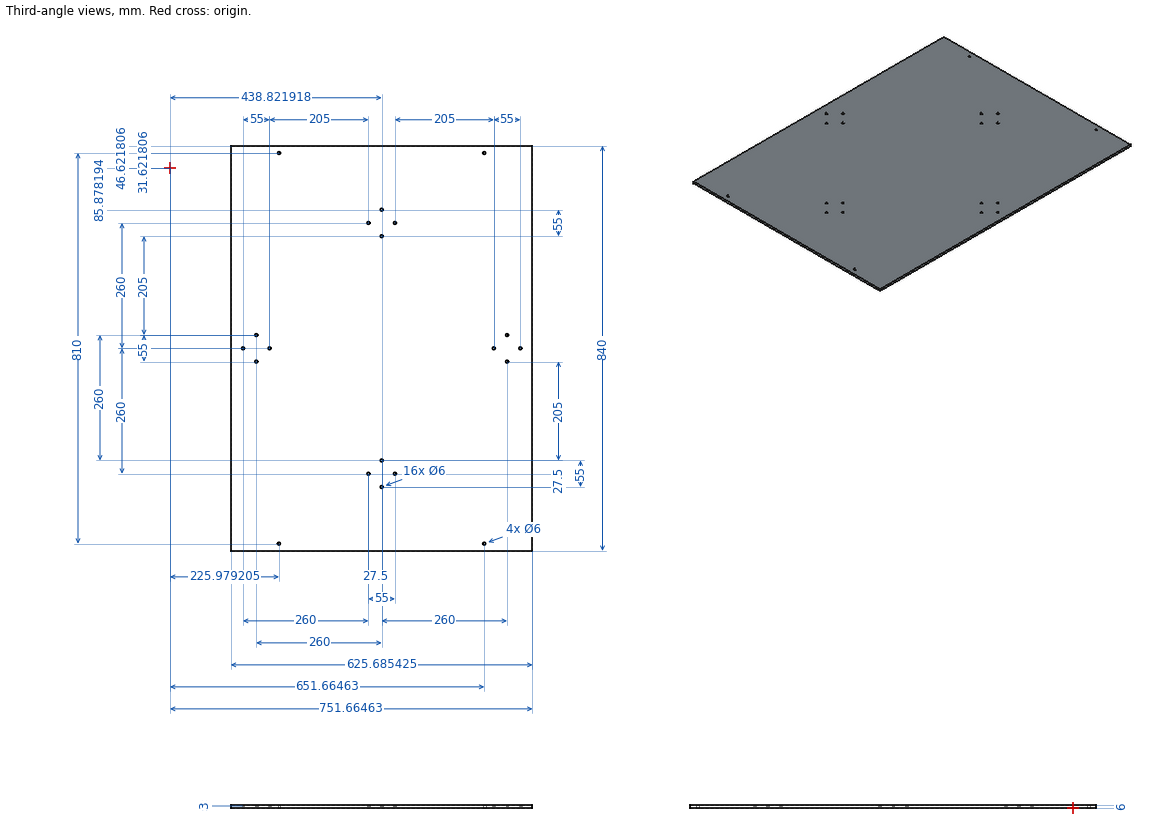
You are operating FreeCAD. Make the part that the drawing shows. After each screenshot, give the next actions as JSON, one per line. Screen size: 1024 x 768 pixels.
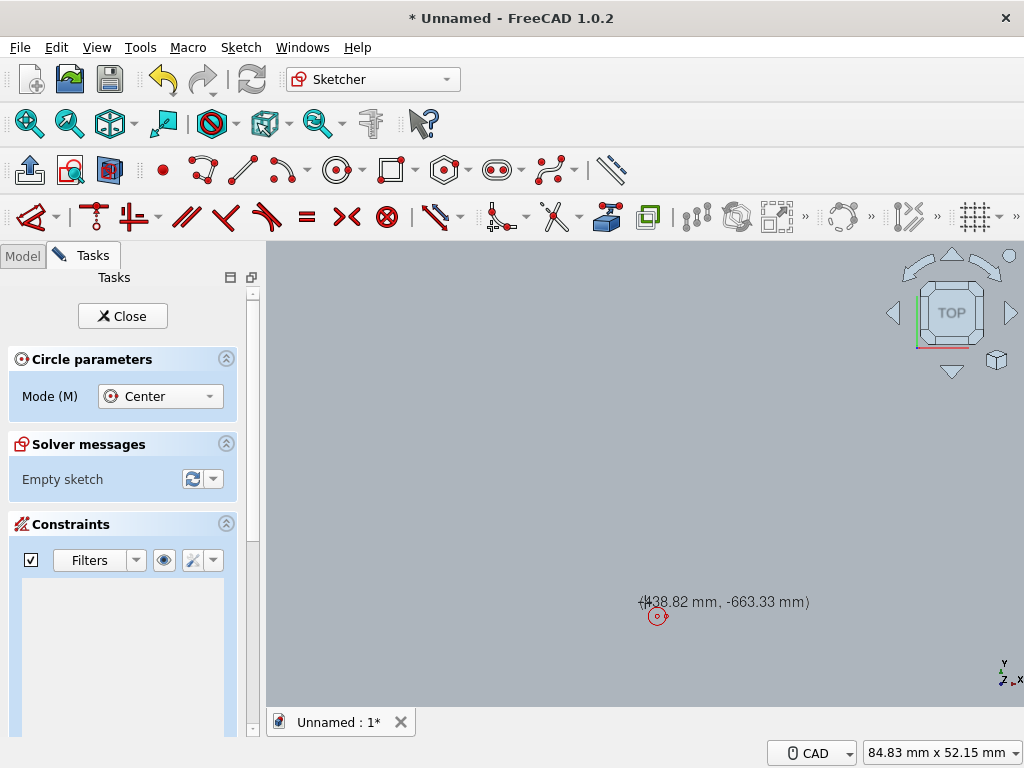
{"action": "scroll", "coordinate": [608, 622], "scroll_direction": "down", "scroll_amount": 15}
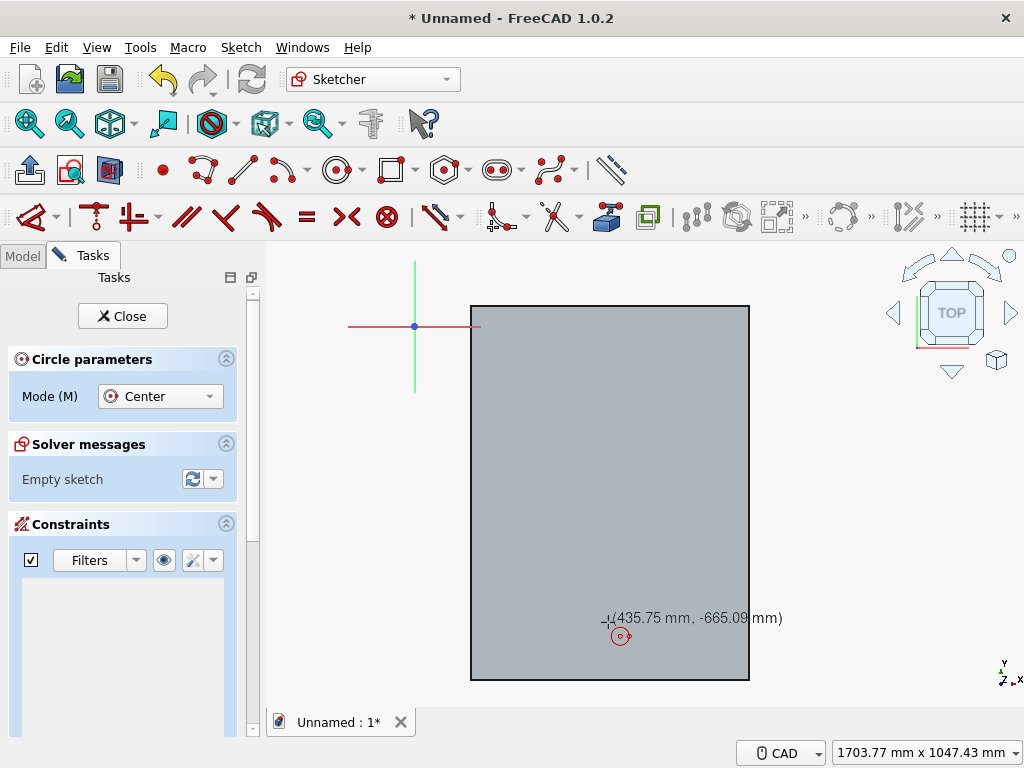
{"action": "left_click", "coordinate": [610, 621]}
{"action": "mouse_move", "coordinate": [611, 620]}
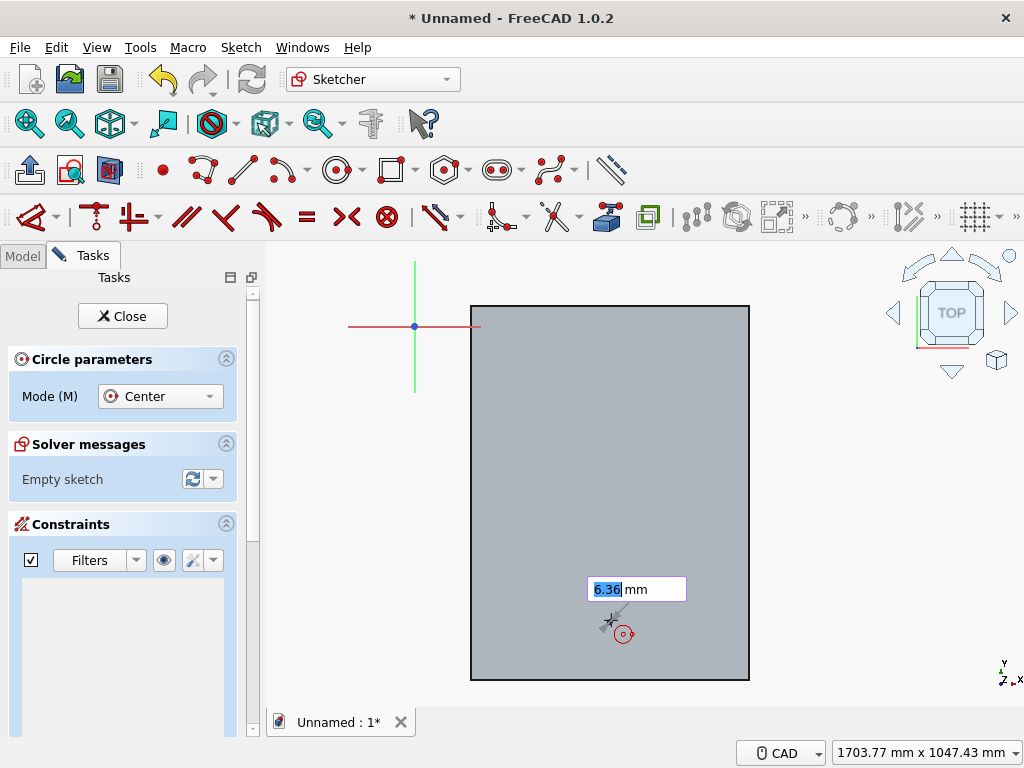
{"action": "type", "text": "6"}
{"action": "key", "text": "Return"}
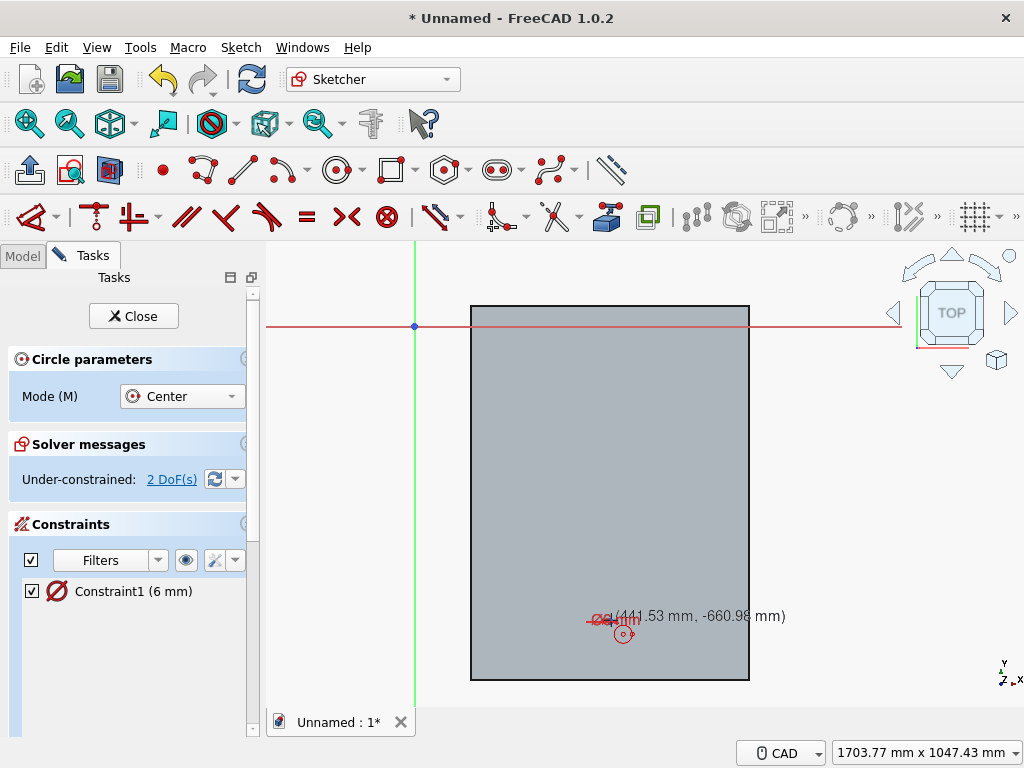
{"action": "scroll", "coordinate": [598, 609], "scroll_direction": "up", "scroll_amount": 15}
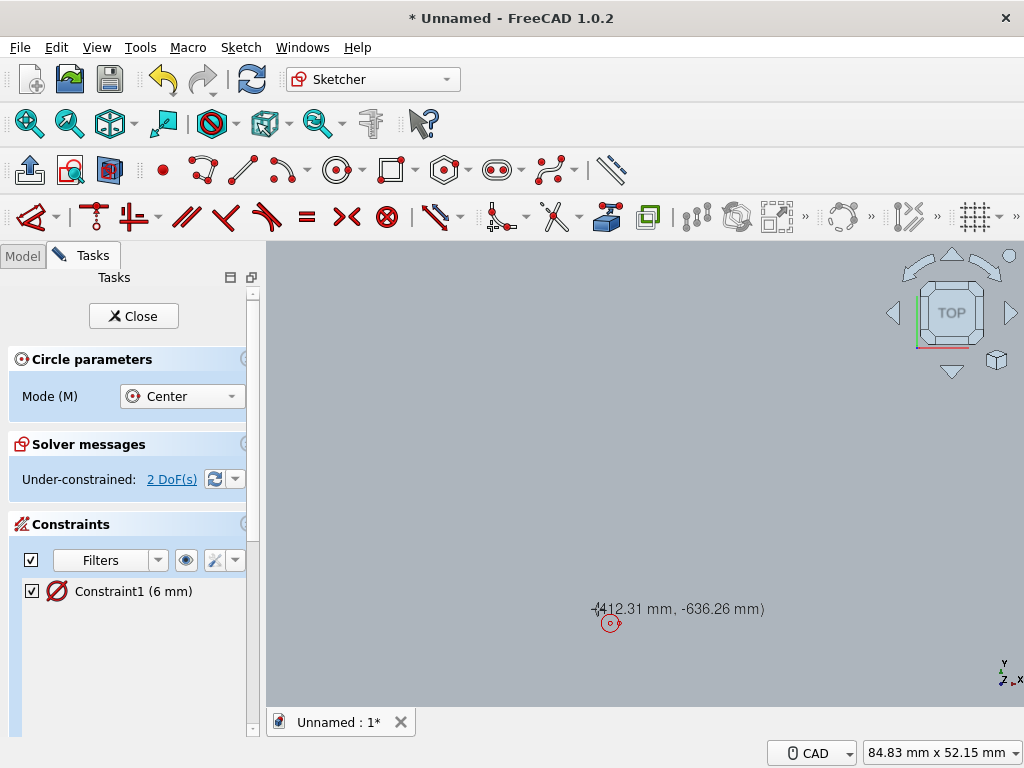
{"action": "scroll", "coordinate": [598, 609], "scroll_direction": "down", "scroll_amount": 15}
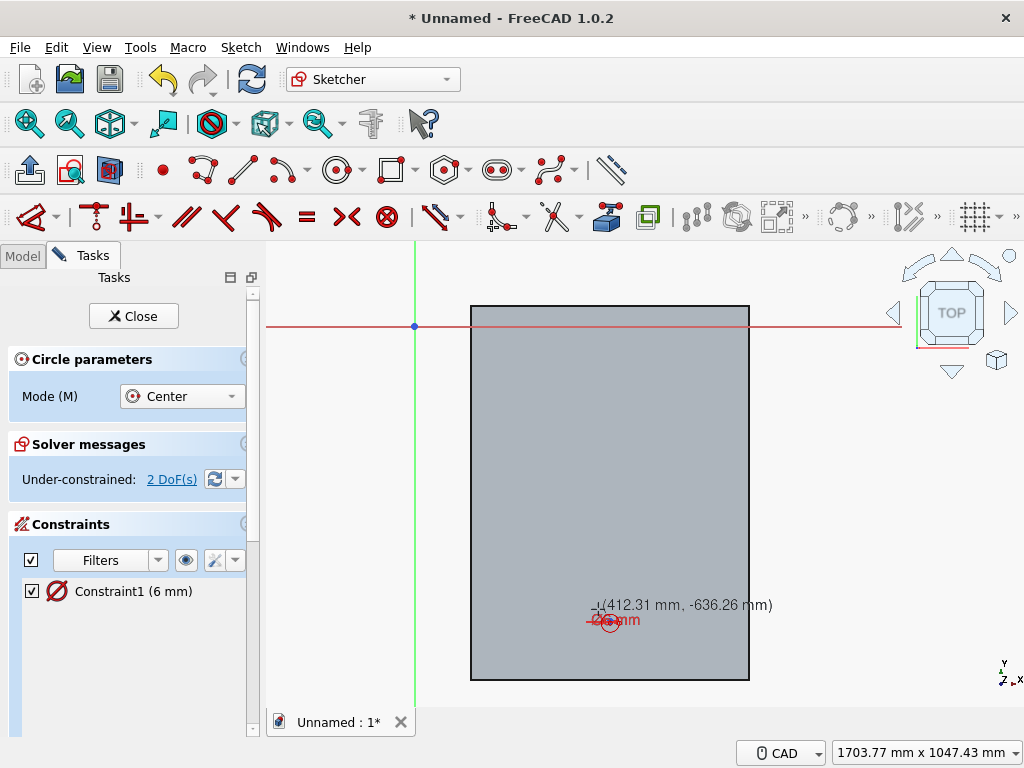
{"action": "left_click", "coordinate": [598, 609]}
{"action": "mouse_move", "coordinate": [599, 608]}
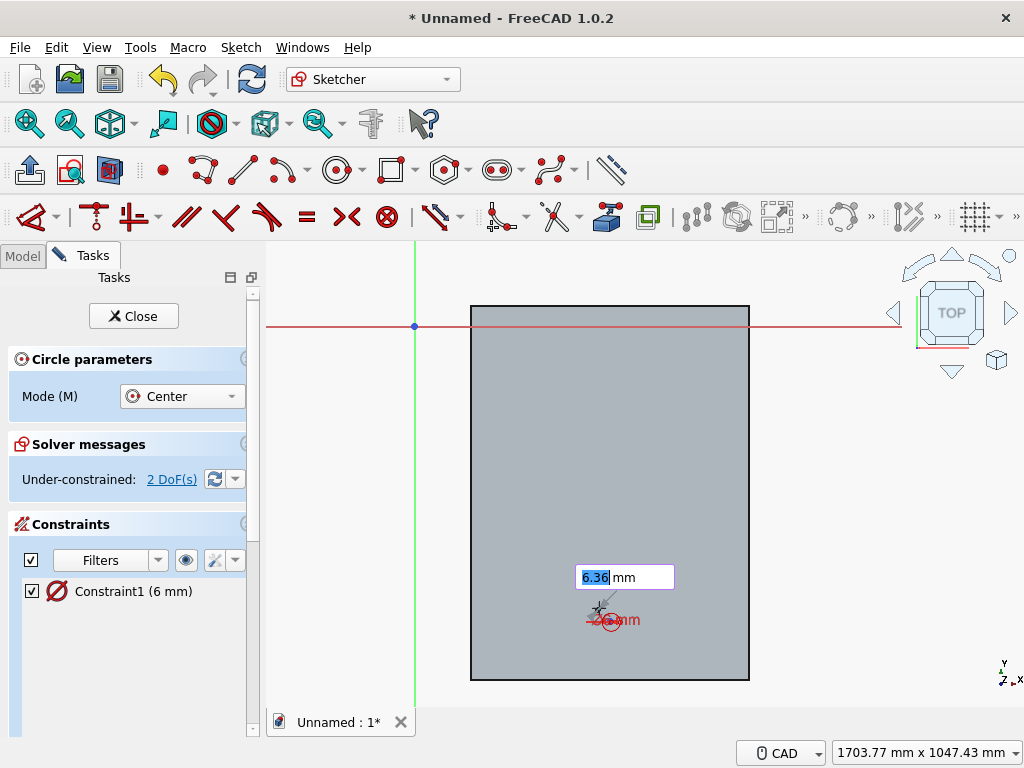
{"action": "type", "text": "6"}
{"action": "key", "text": "Return"}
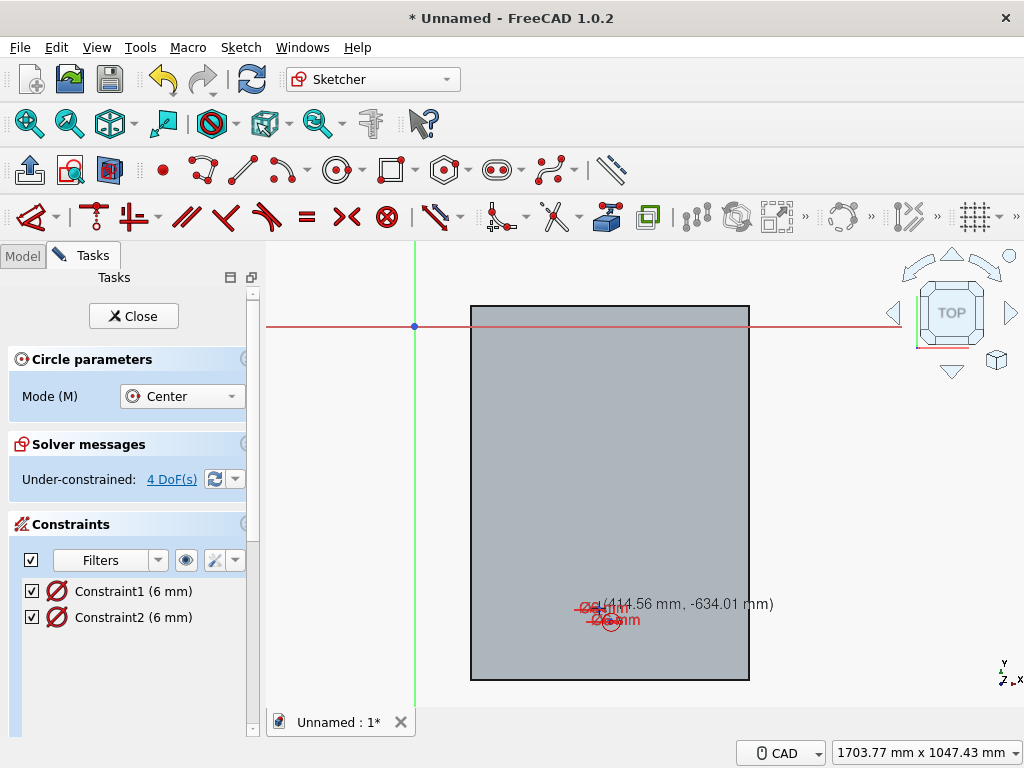
{"action": "scroll", "coordinate": [610, 596], "scroll_direction": "up", "scroll_amount": 15}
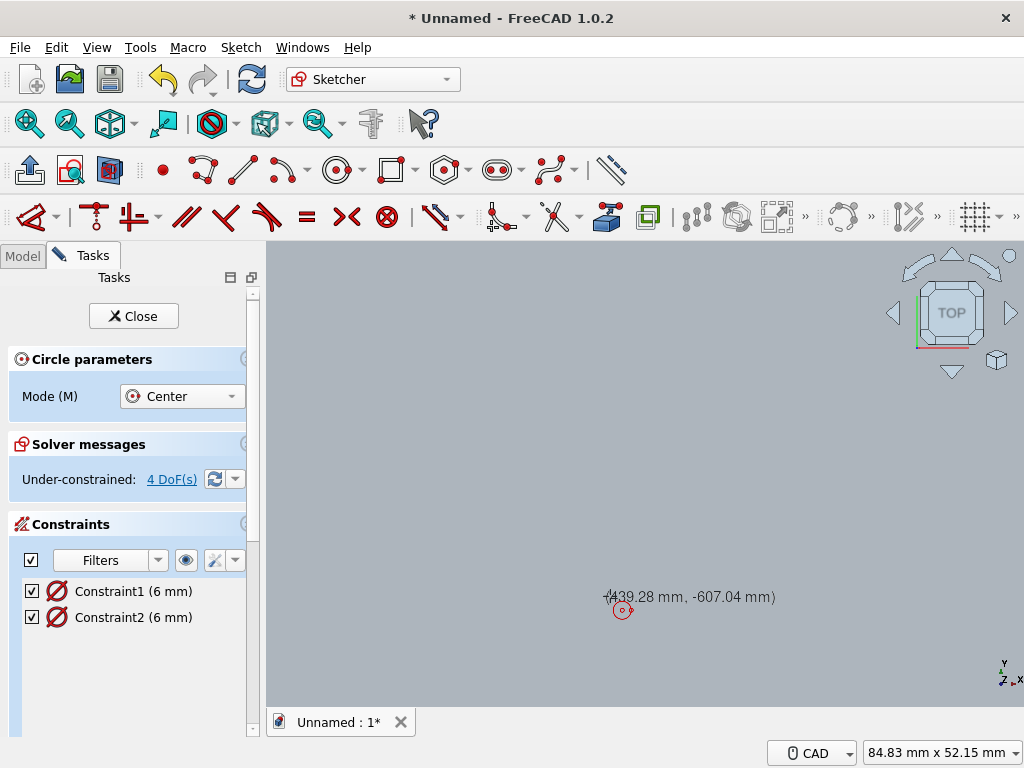
{"action": "scroll", "coordinate": [610, 596], "scroll_direction": "down", "scroll_amount": 15}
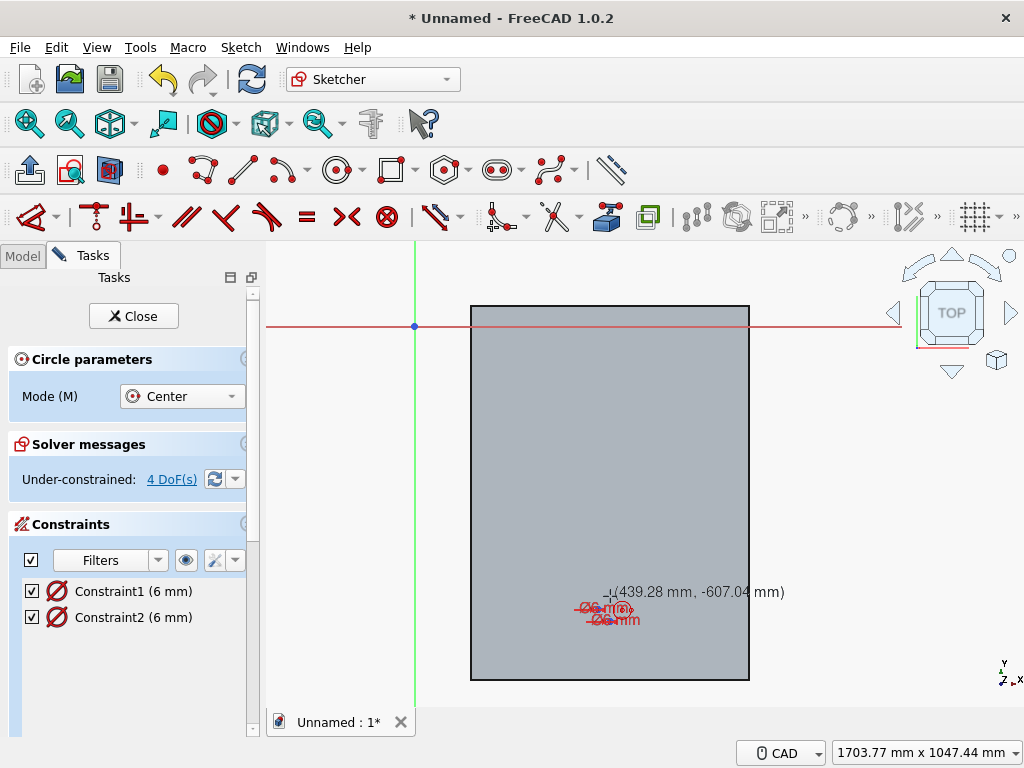
{"action": "left_click", "coordinate": [610, 596]}
{"action": "mouse_move", "coordinate": [611, 596]}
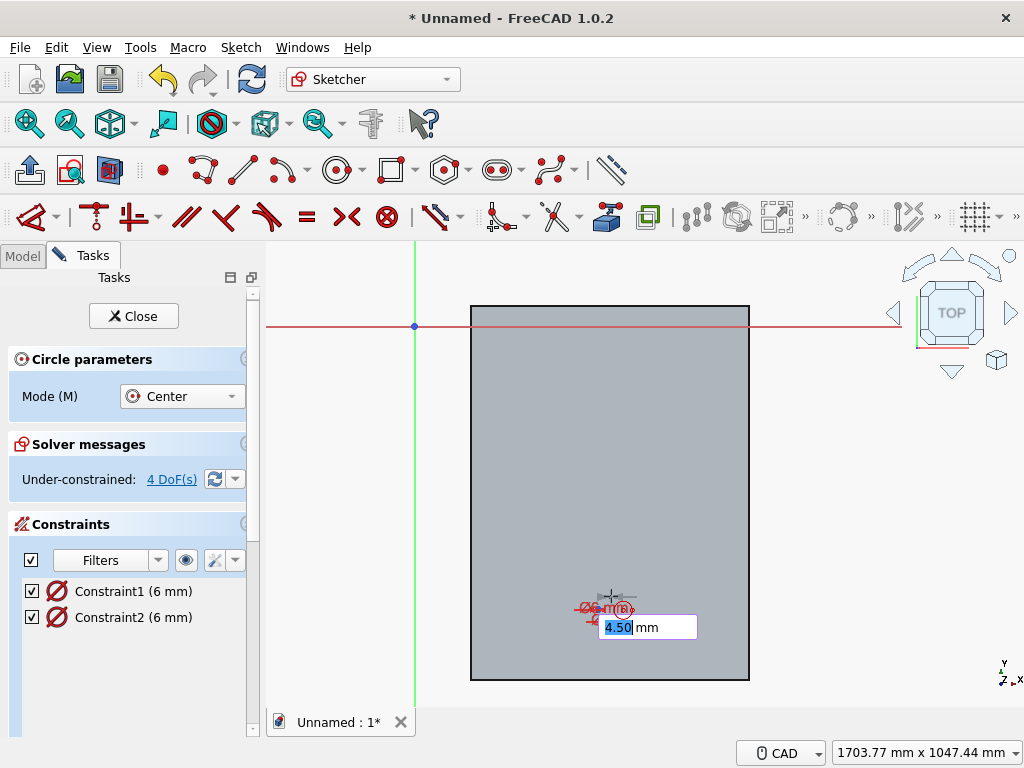
{"action": "type", "text": "6"}
{"action": "key", "text": "Return"}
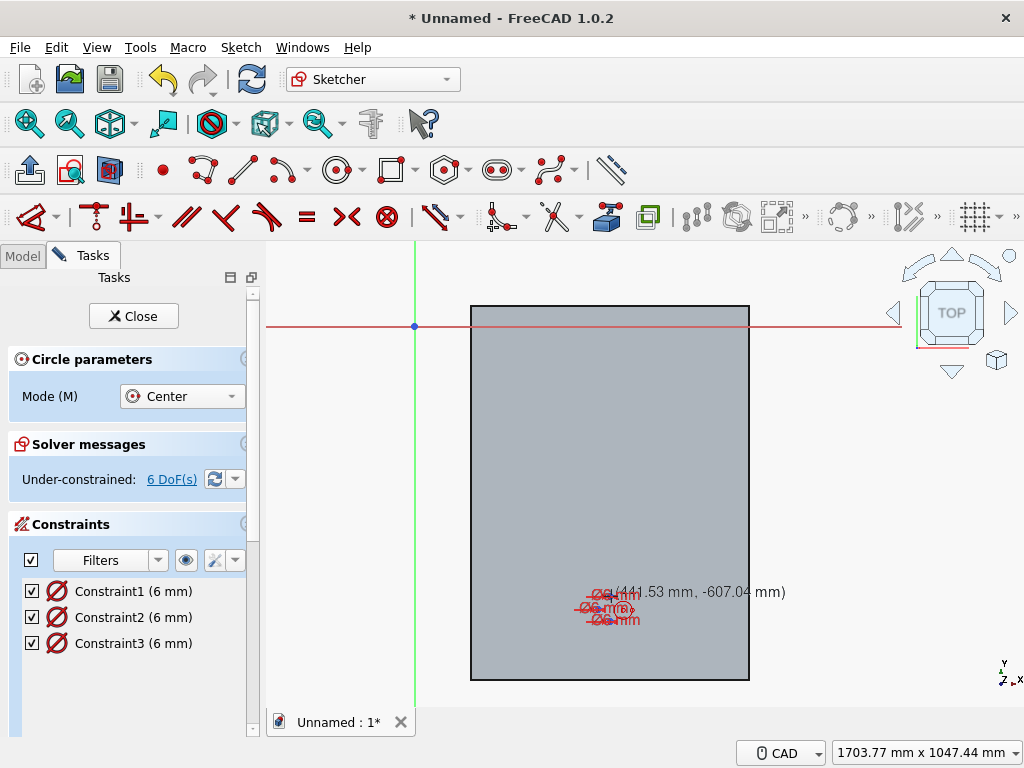
{"action": "scroll", "coordinate": [622, 609], "scroll_direction": "up", "scroll_amount": 15}